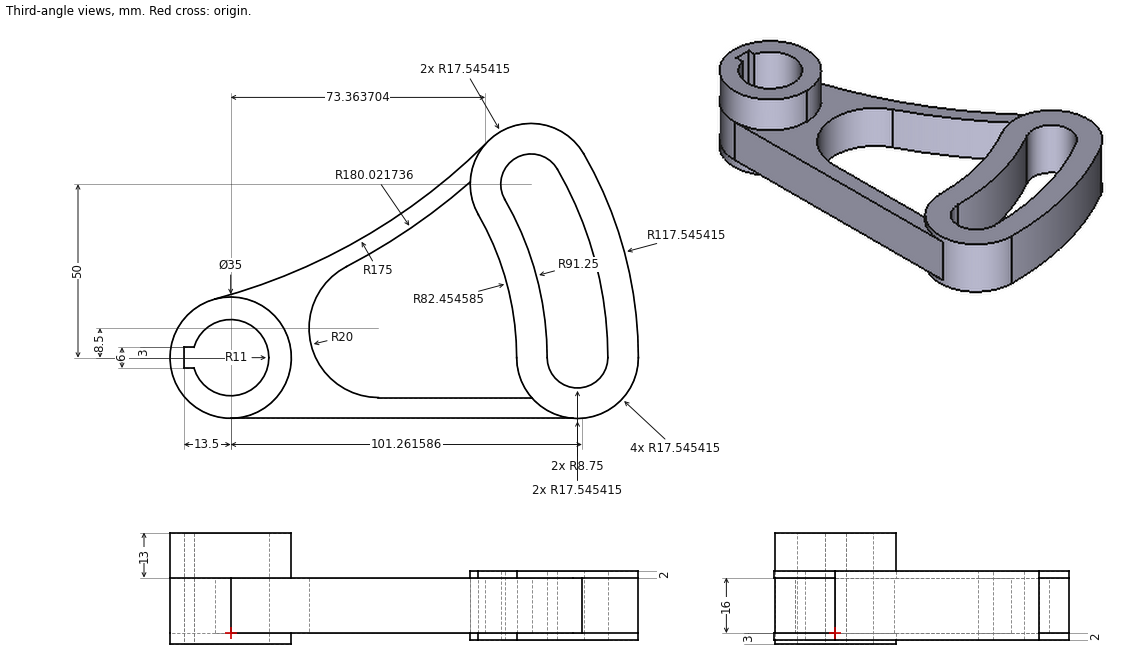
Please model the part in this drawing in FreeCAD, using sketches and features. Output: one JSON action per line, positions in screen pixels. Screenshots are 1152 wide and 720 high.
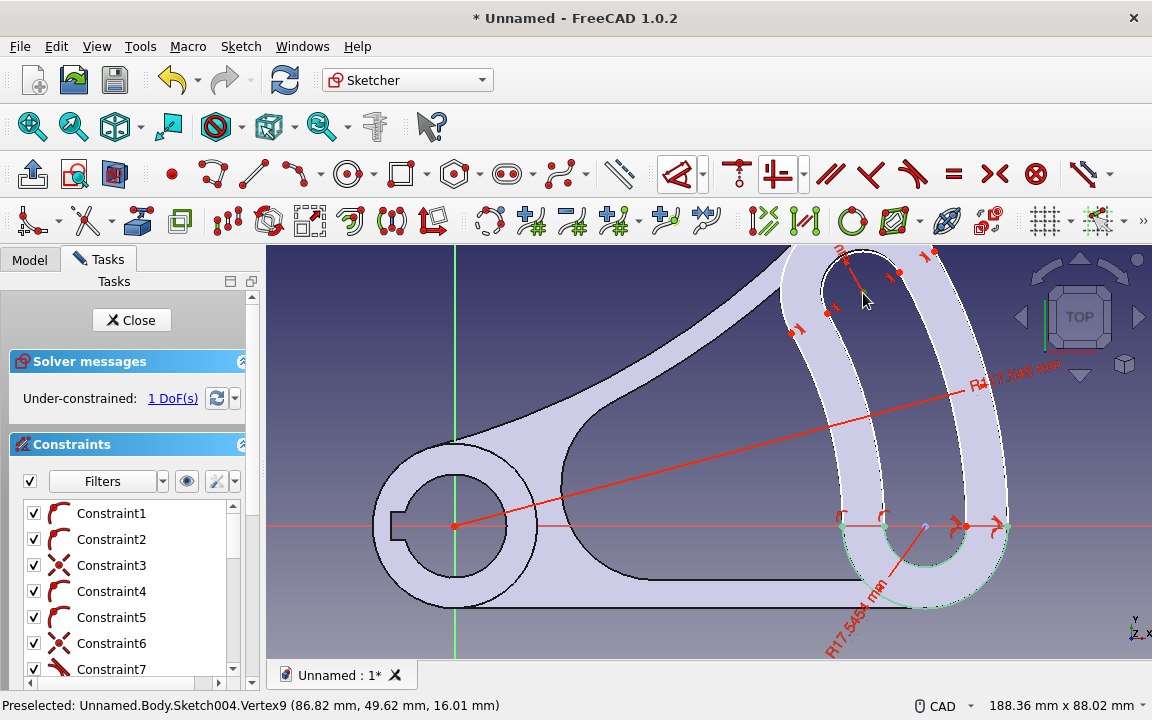
{"action": "left_click", "coordinate": [702, 174]}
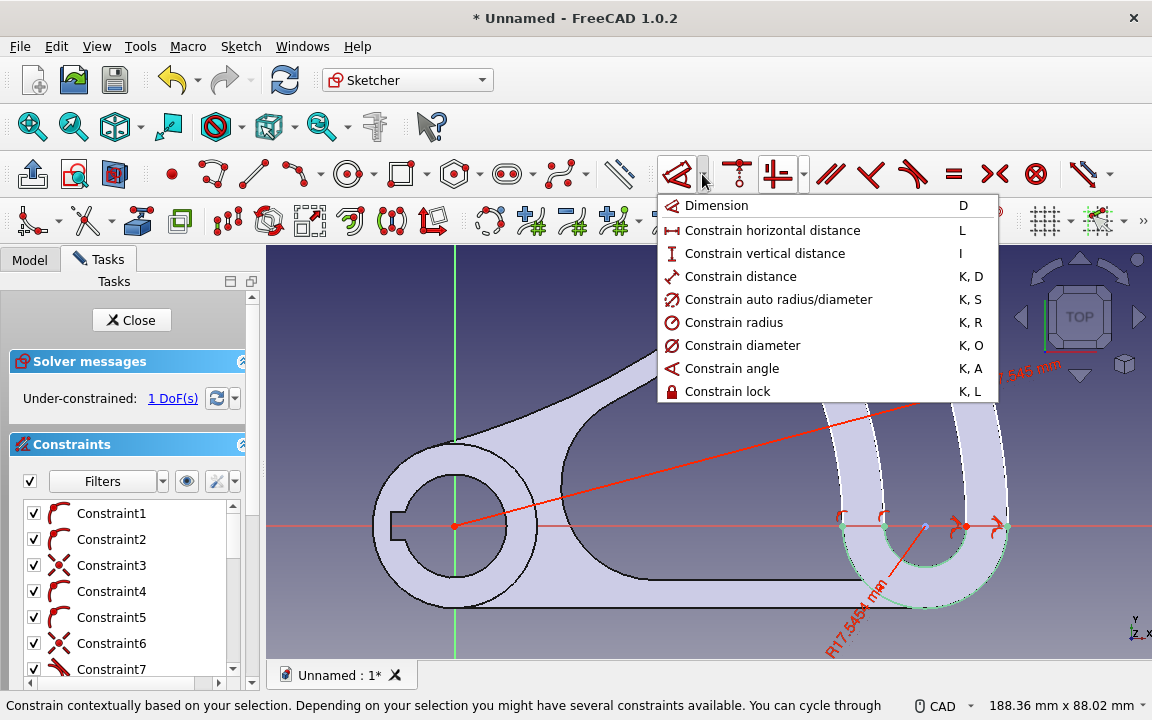
{"action": "left_click", "coordinate": [828, 254]}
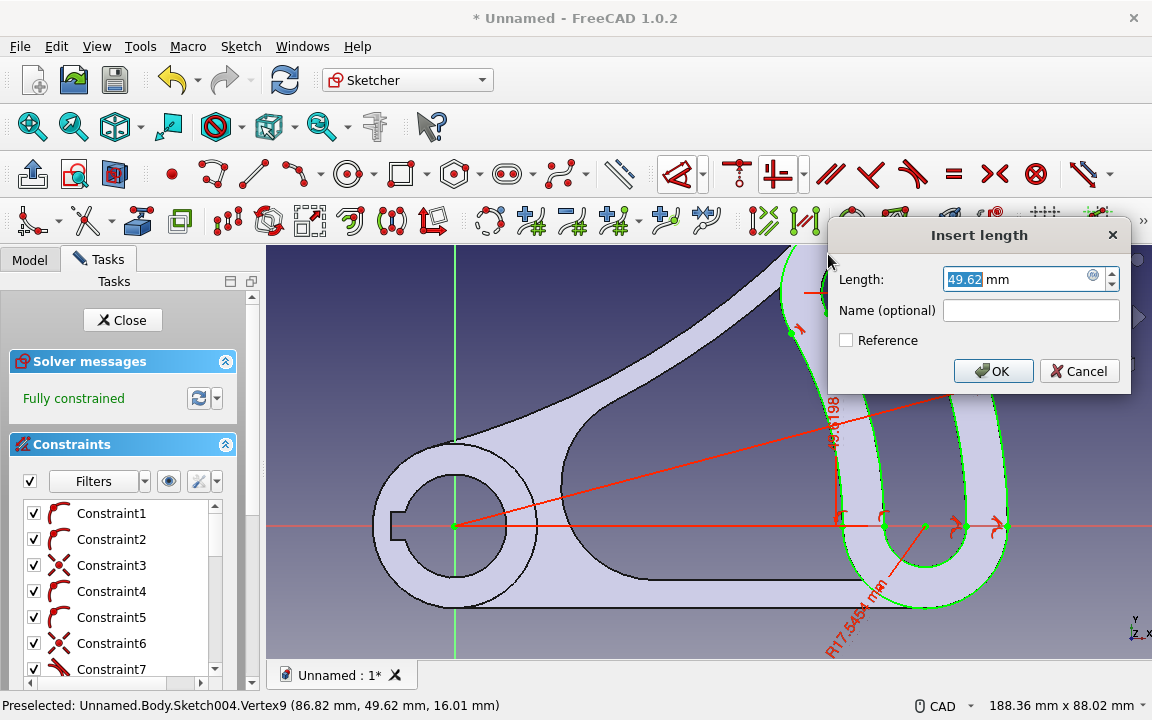
{"action": "type", "text": "50"}
{"action": "key", "text": "Return"}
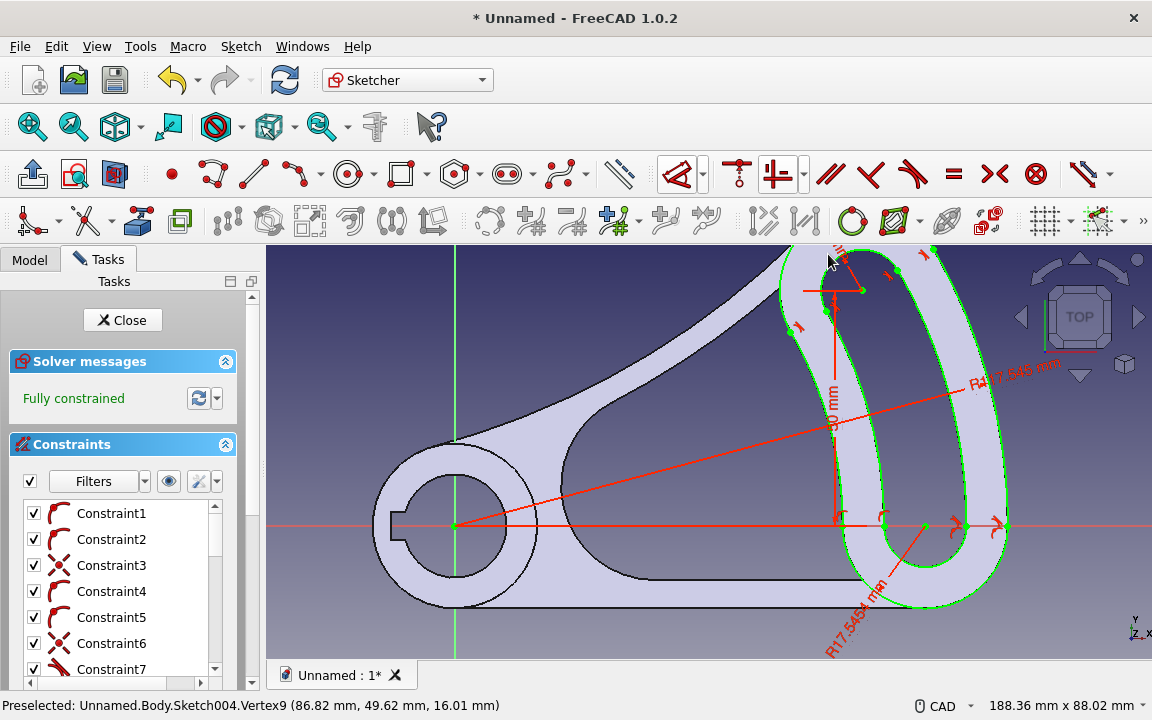
{"action": "left_click", "coordinate": [123, 320]}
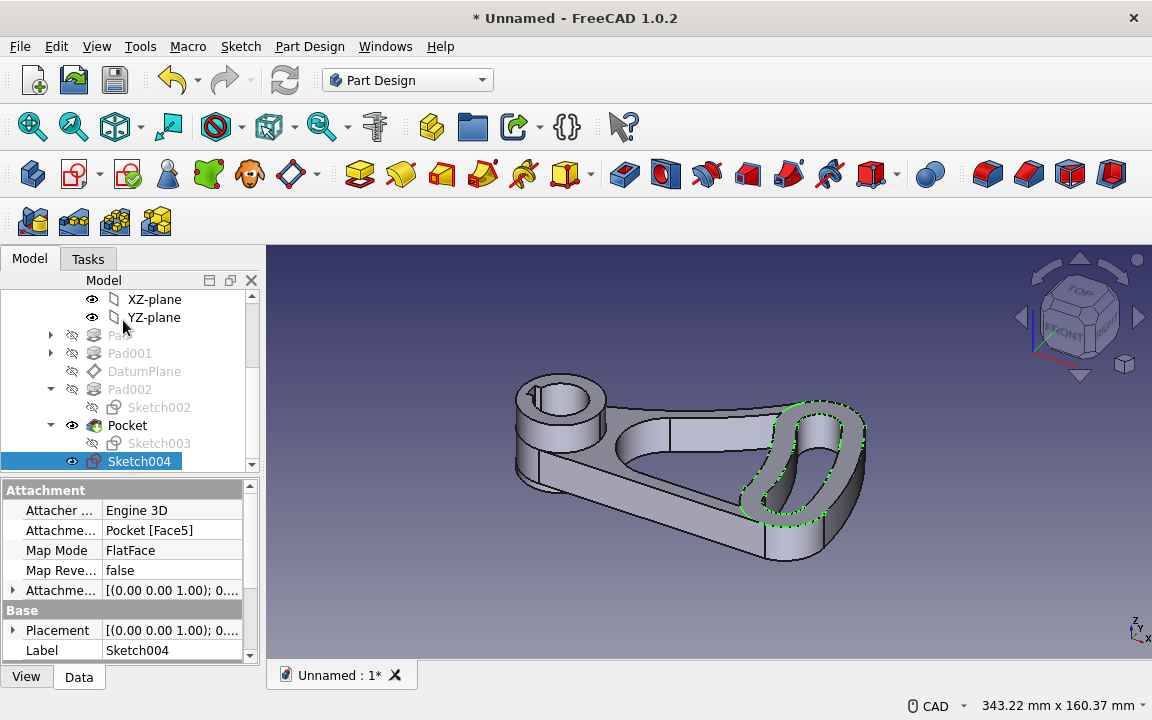
{"action": "left_click", "coordinate": [360, 174]}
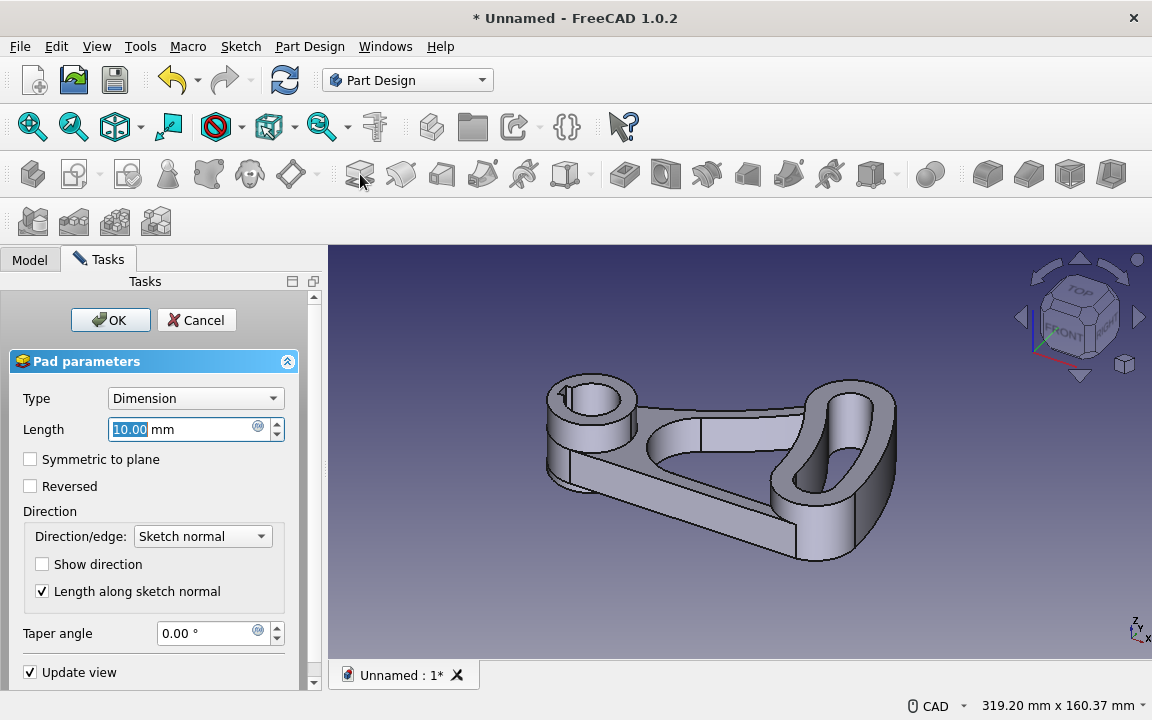
{"action": "type", "text": "2"}
{"action": "key", "text": "Tab"}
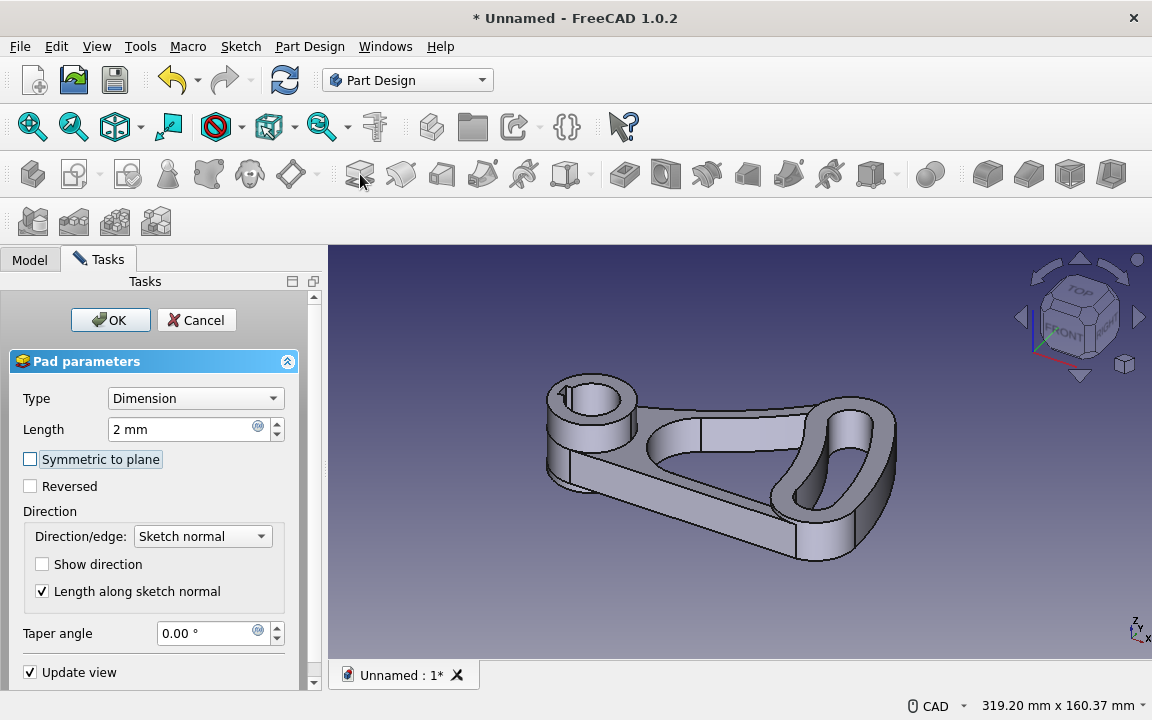
{"action": "left_click", "coordinate": [111, 320]}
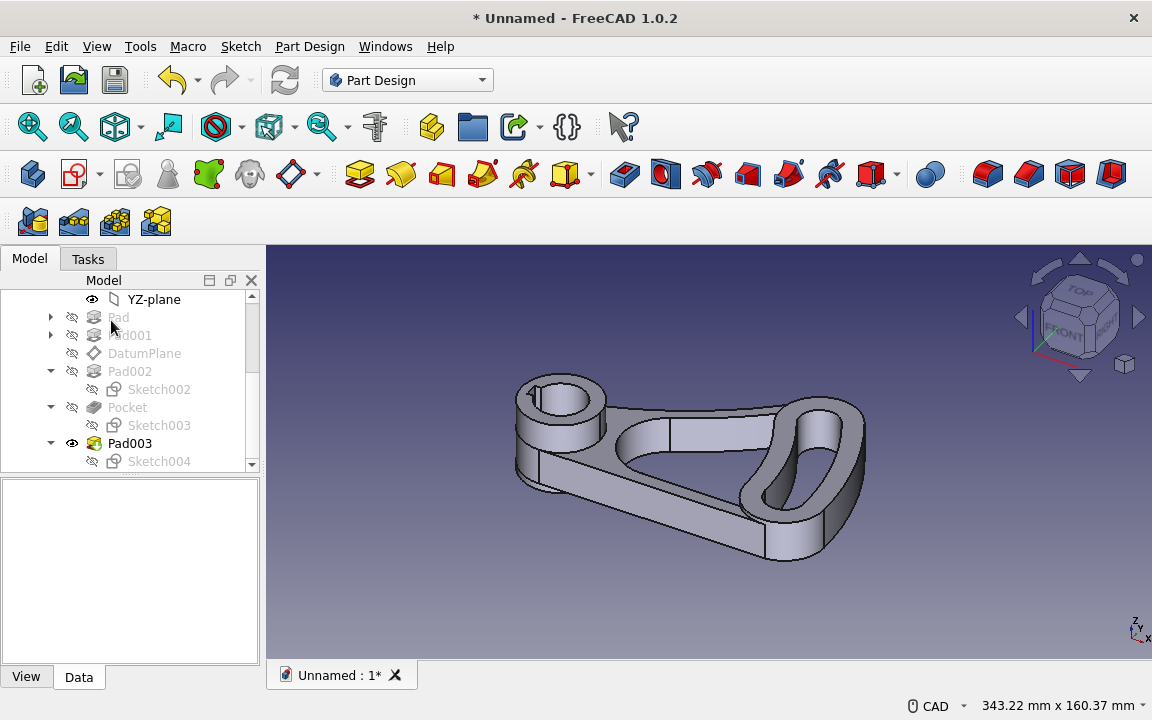
{"action": "scroll", "coordinate": [161, 385], "scroll_direction": "down", "scroll_amount": 3}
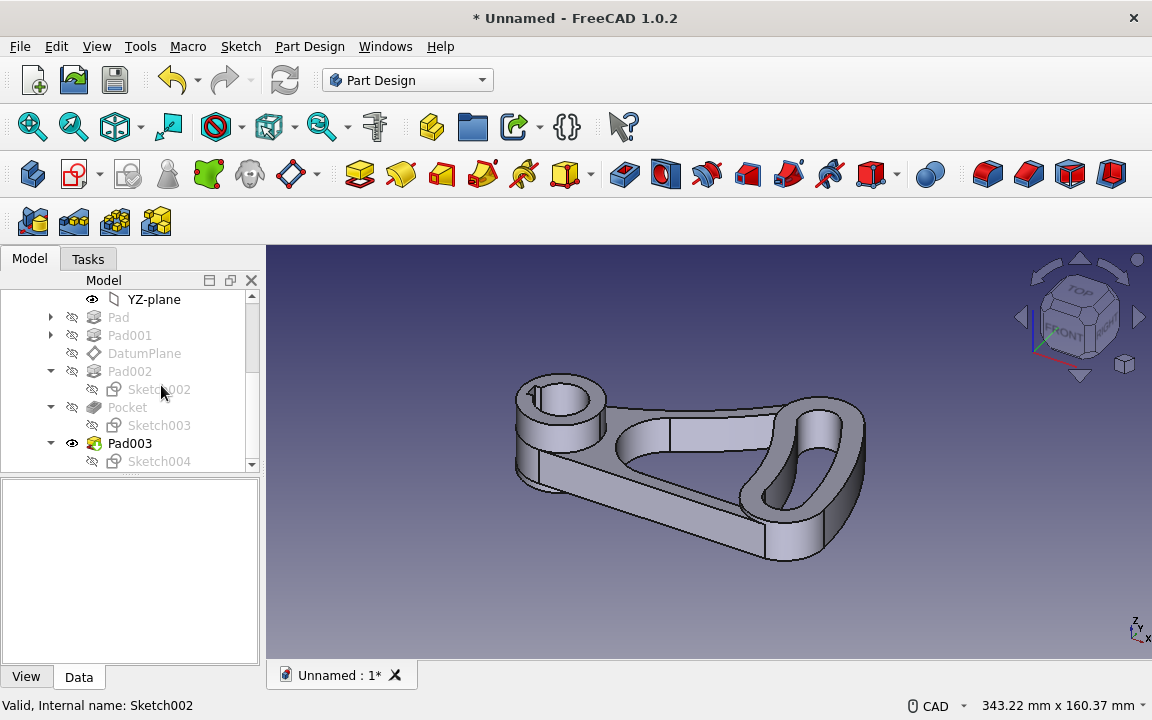
{"action": "scroll", "coordinate": [161, 385], "scroll_direction": "up", "scroll_amount": 15}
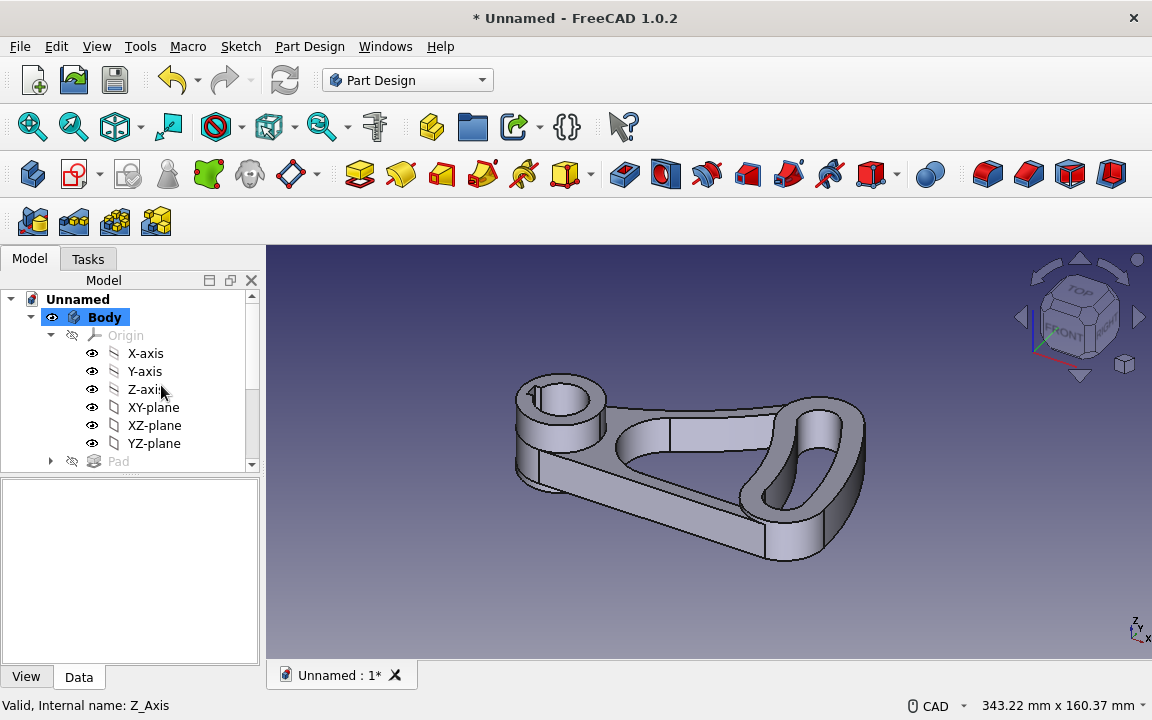
{"action": "left_click", "coordinate": [137, 407]}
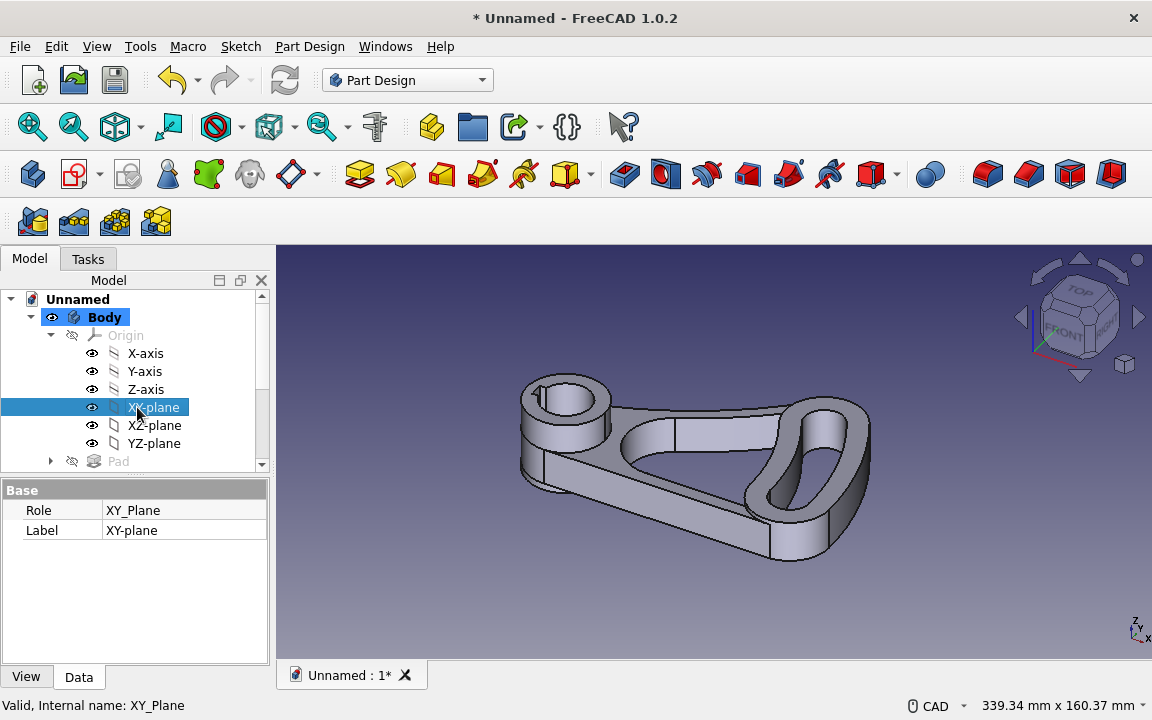
{"action": "left_click", "coordinate": [290, 174]}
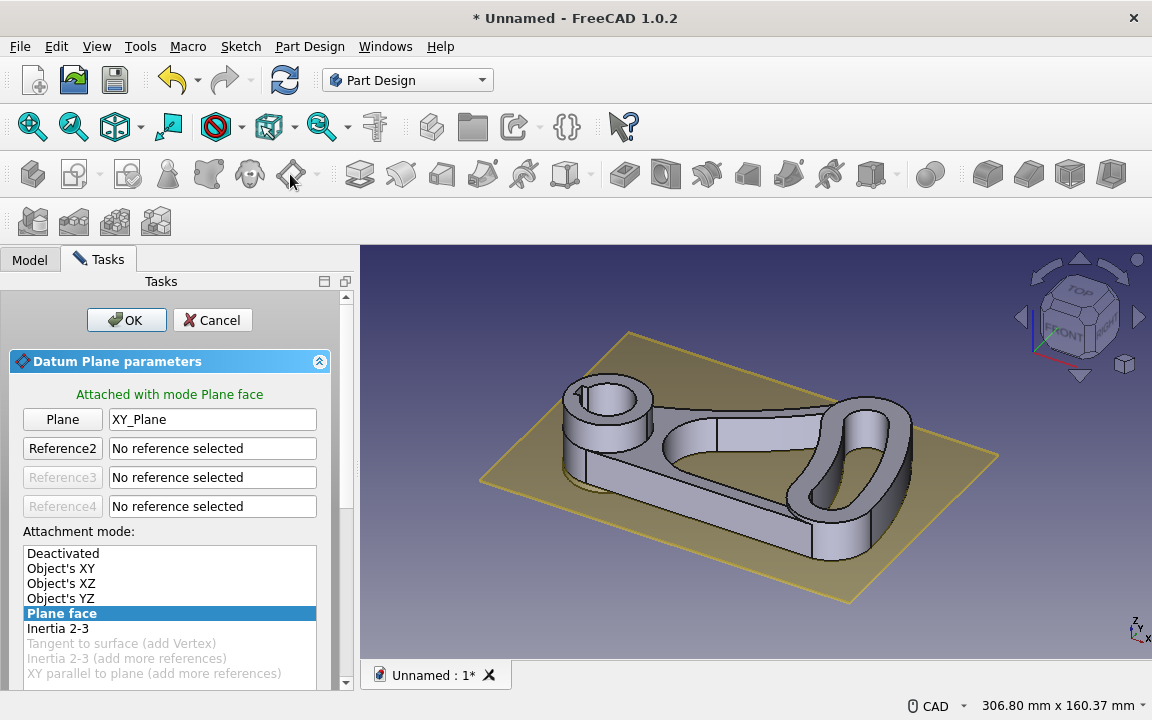
{"action": "scroll", "coordinate": [346, 490], "scroll_direction": "down", "scroll_amount": 4}